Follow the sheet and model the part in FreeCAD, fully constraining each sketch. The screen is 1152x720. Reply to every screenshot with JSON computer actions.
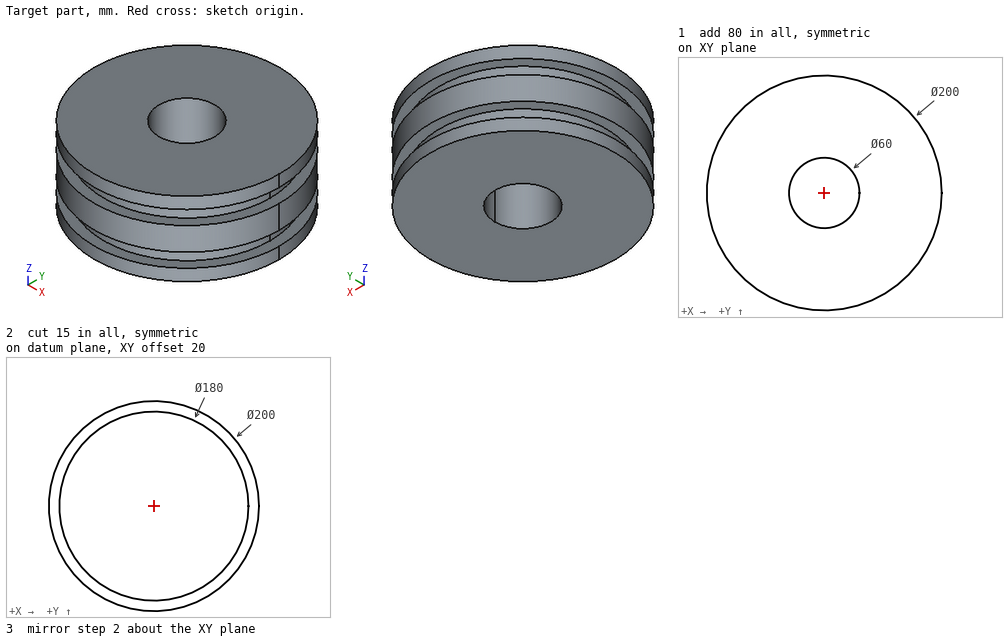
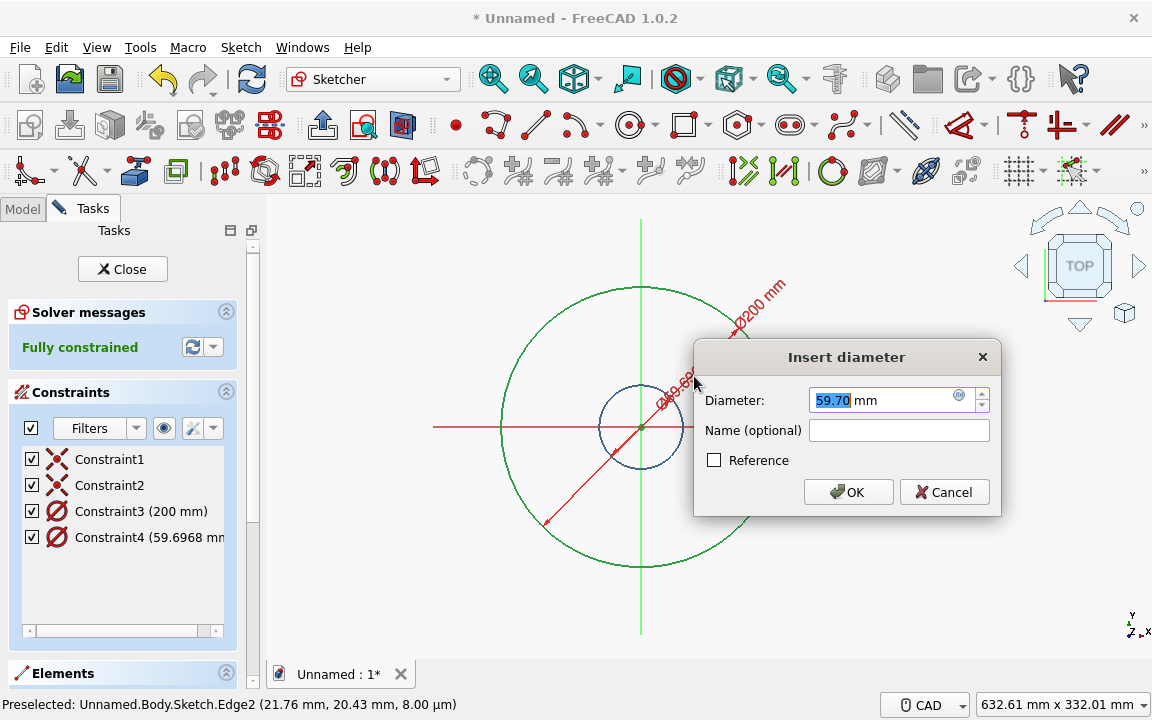
{"action": "type", "text": "60"}
{"action": "key", "text": "Return"}
{"action": "key", "text": "Escape"}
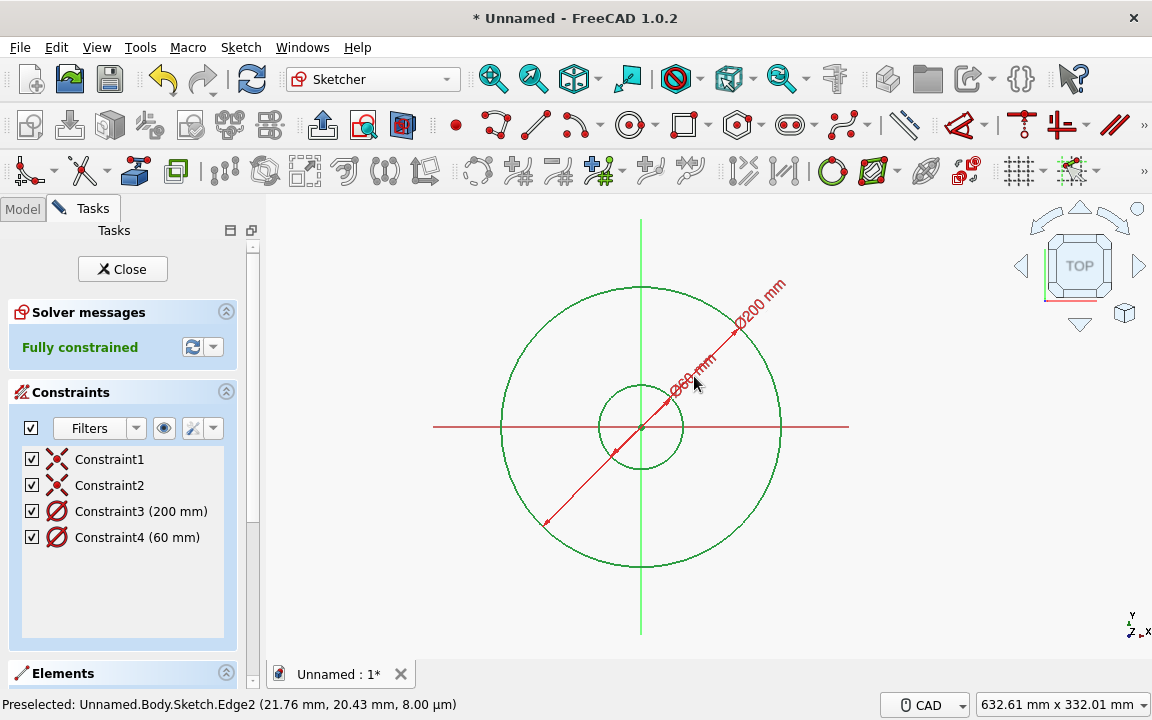
{"action": "left_click", "coordinate": [123, 269]}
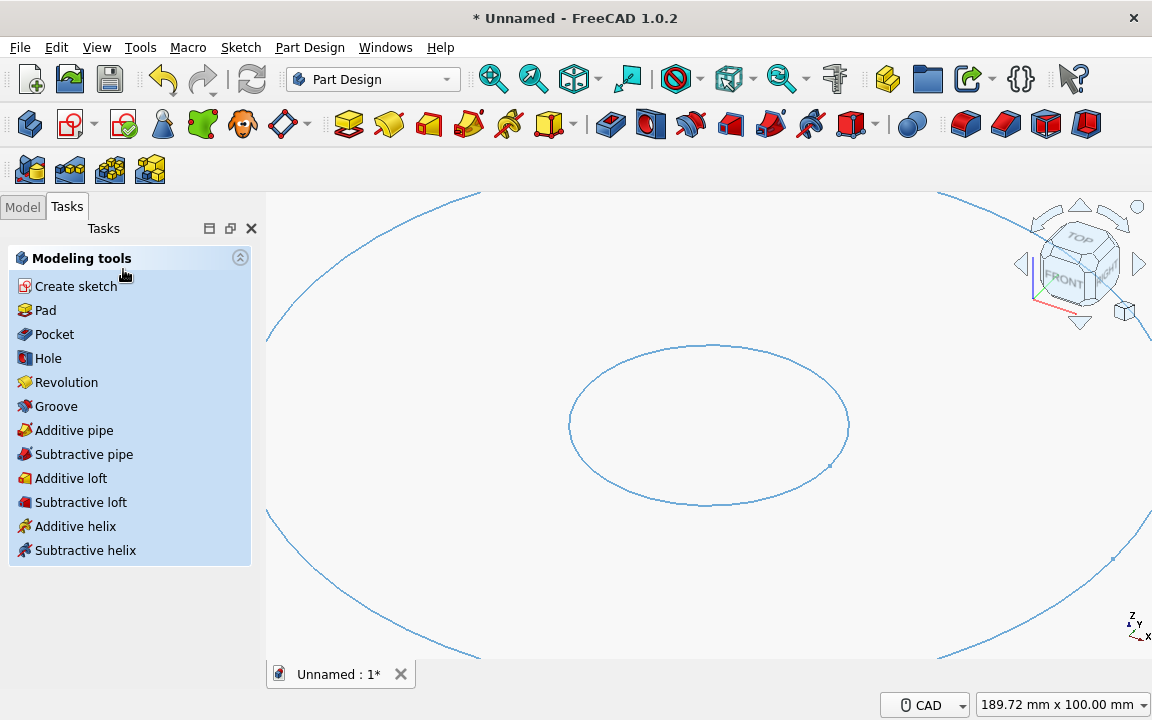
{"action": "left_click", "coordinate": [350, 124]}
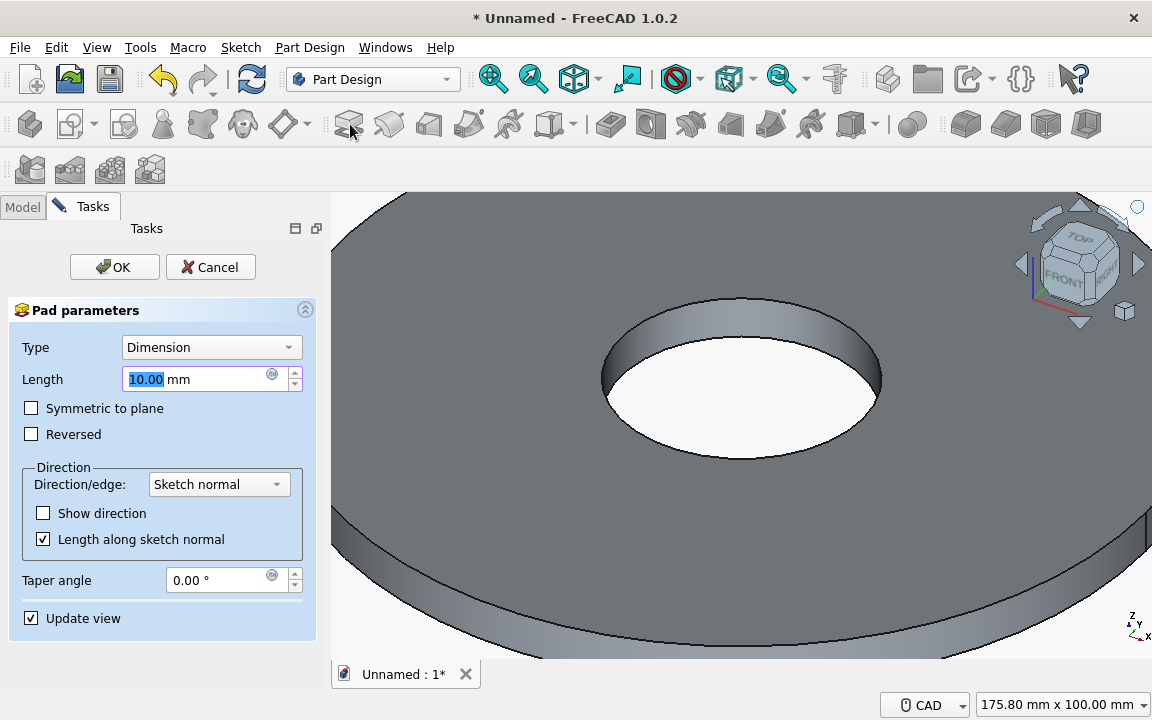
{"action": "type", "text": "80"}
{"action": "key", "text": "Tab"}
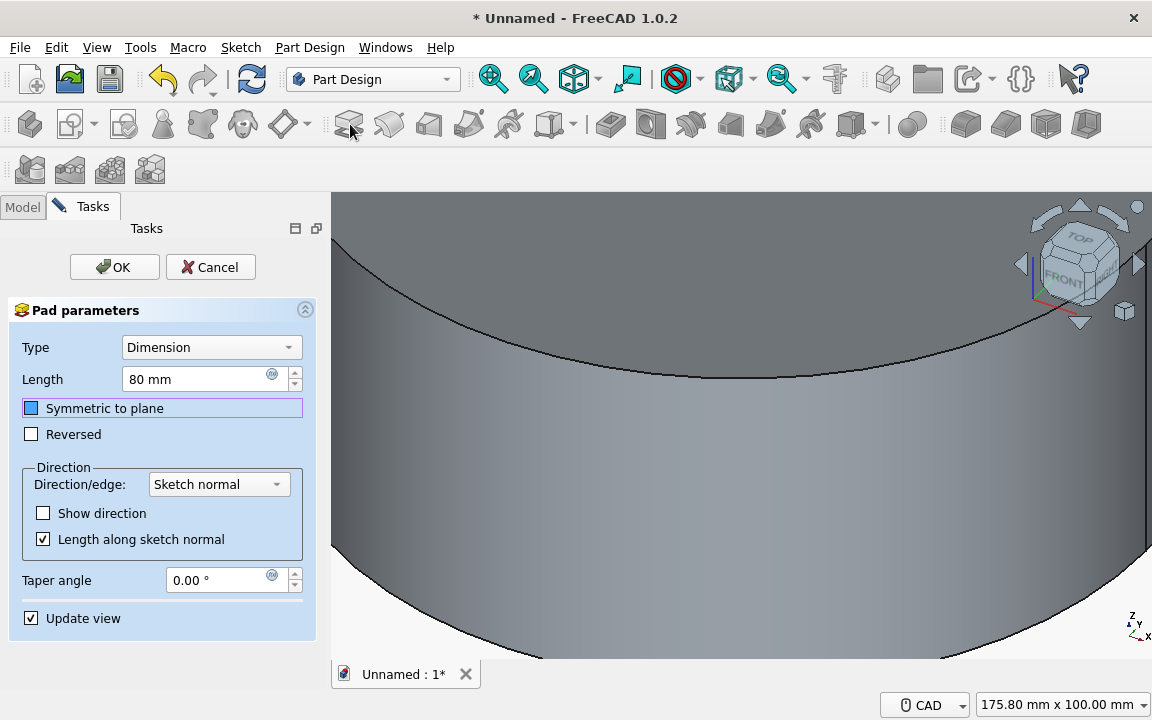
{"action": "left_click", "coordinate": [30, 408]}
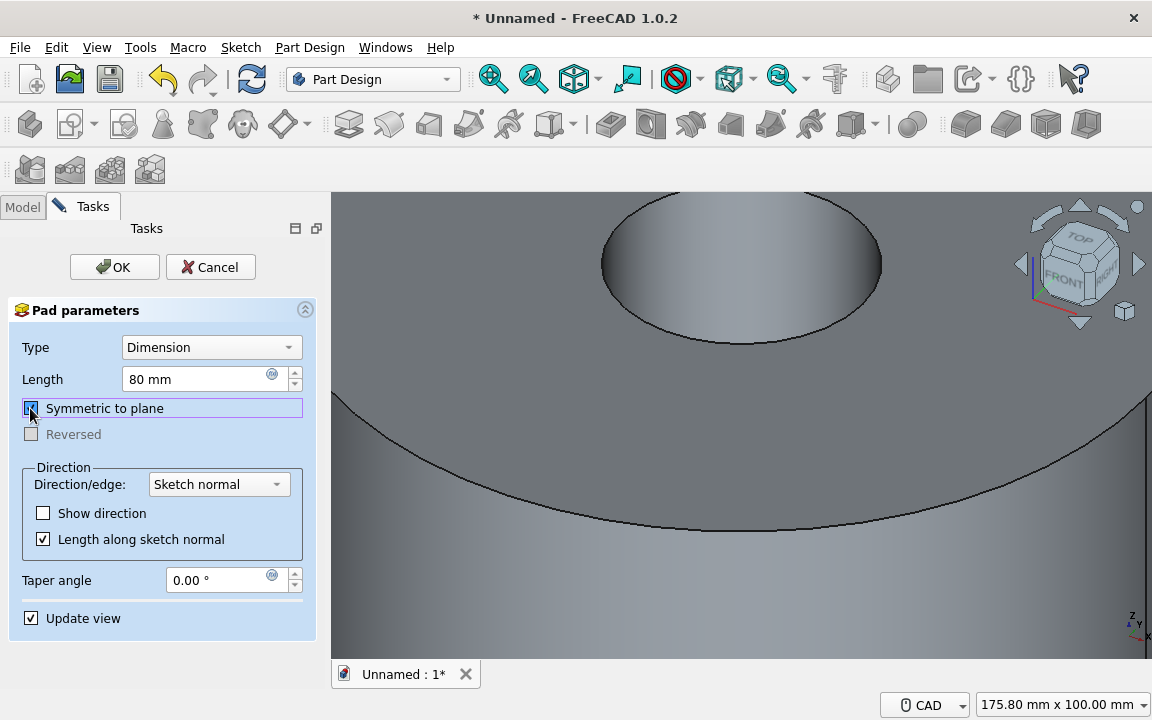
{"action": "left_click", "coordinate": [115, 267]}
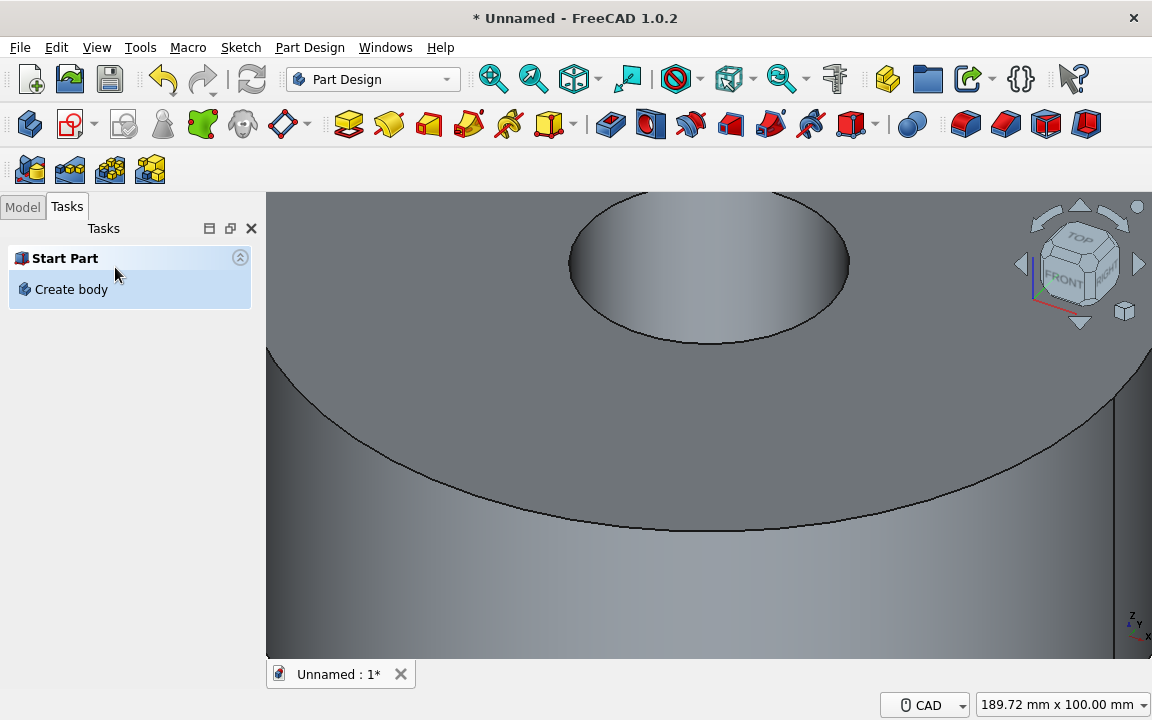
{"action": "left_click", "coordinate": [494, 80]}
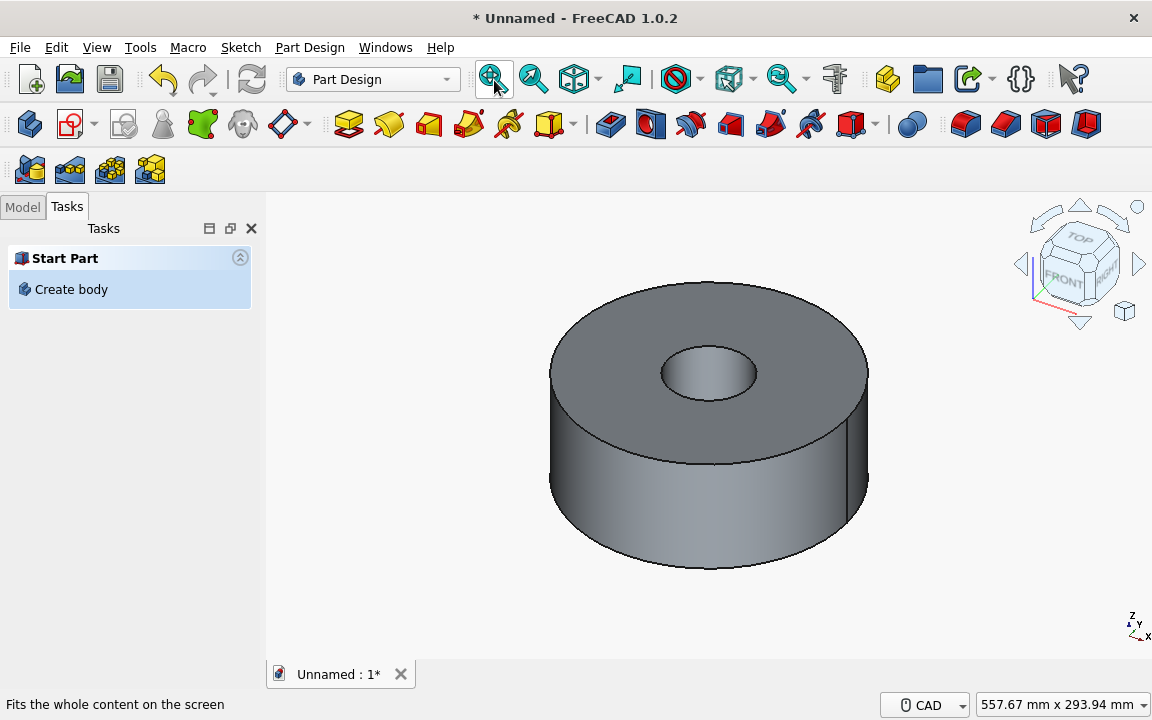
{"action": "left_click", "coordinate": [23, 206]}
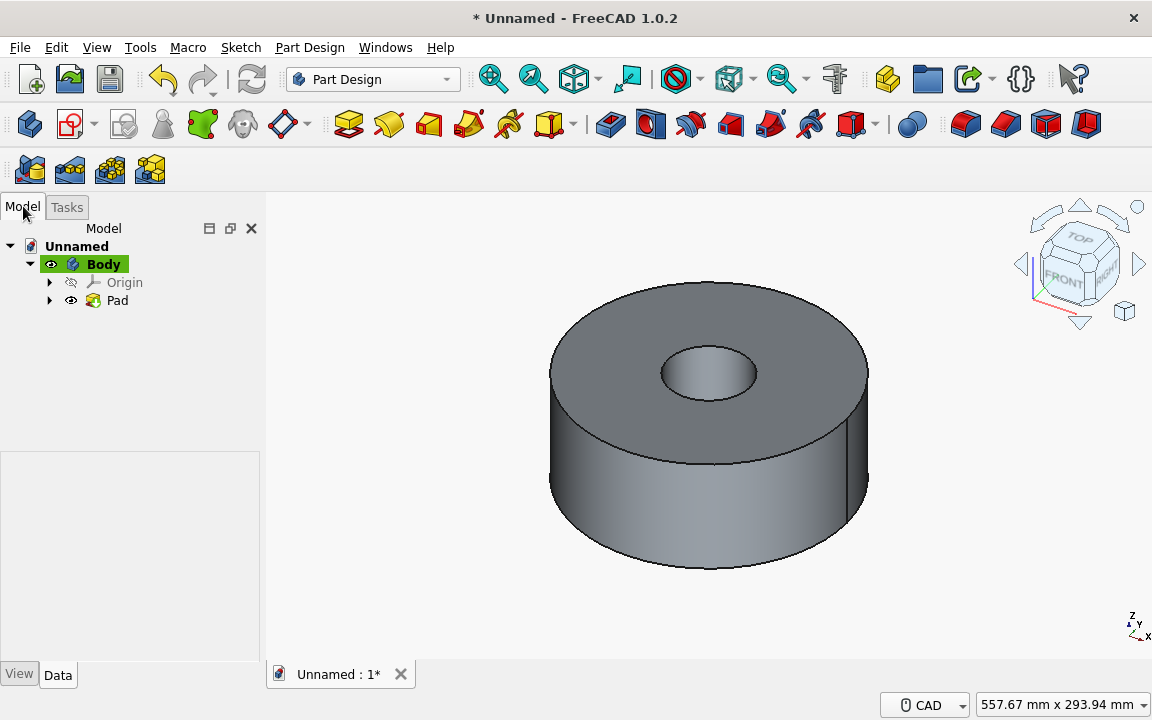
{"action": "left_click", "coordinate": [50, 282]}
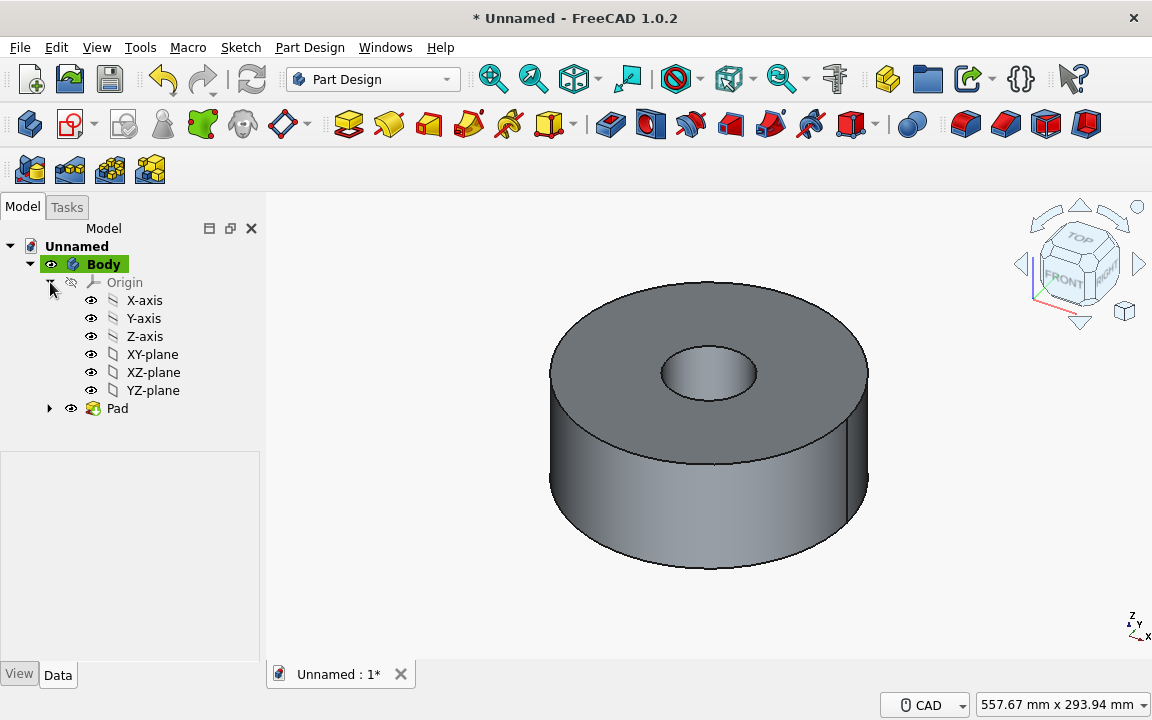
{"action": "left_click", "coordinate": [136, 354]}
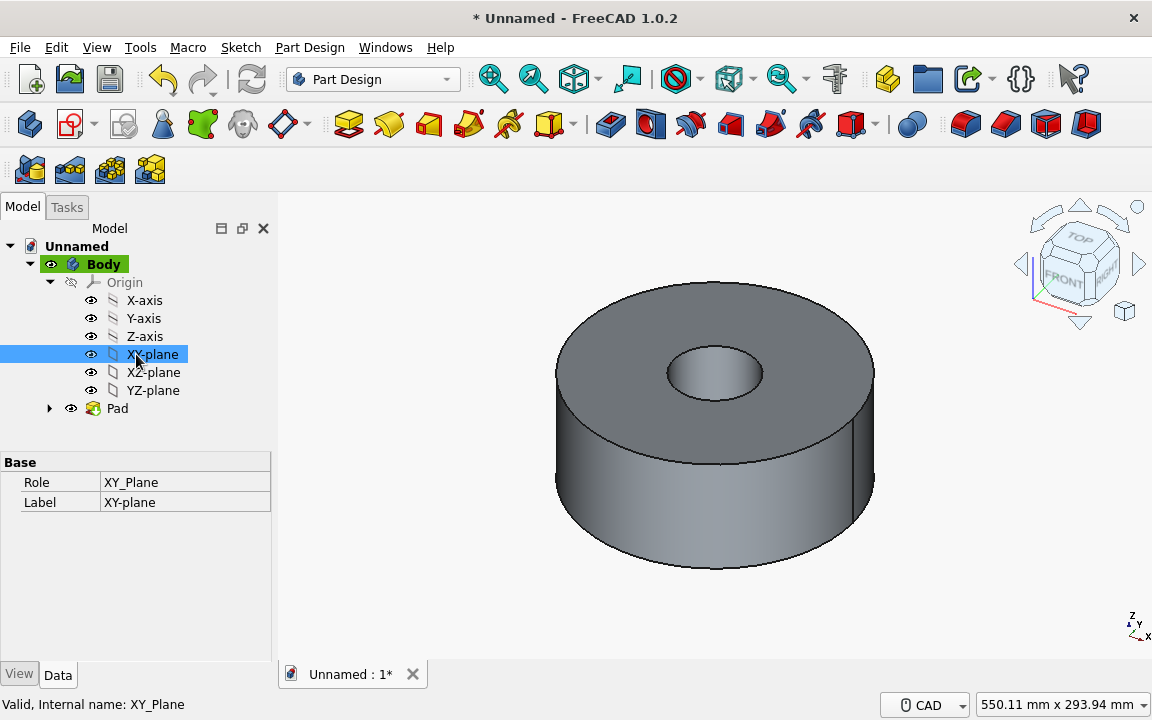
{"action": "left_click", "coordinate": [284, 124]}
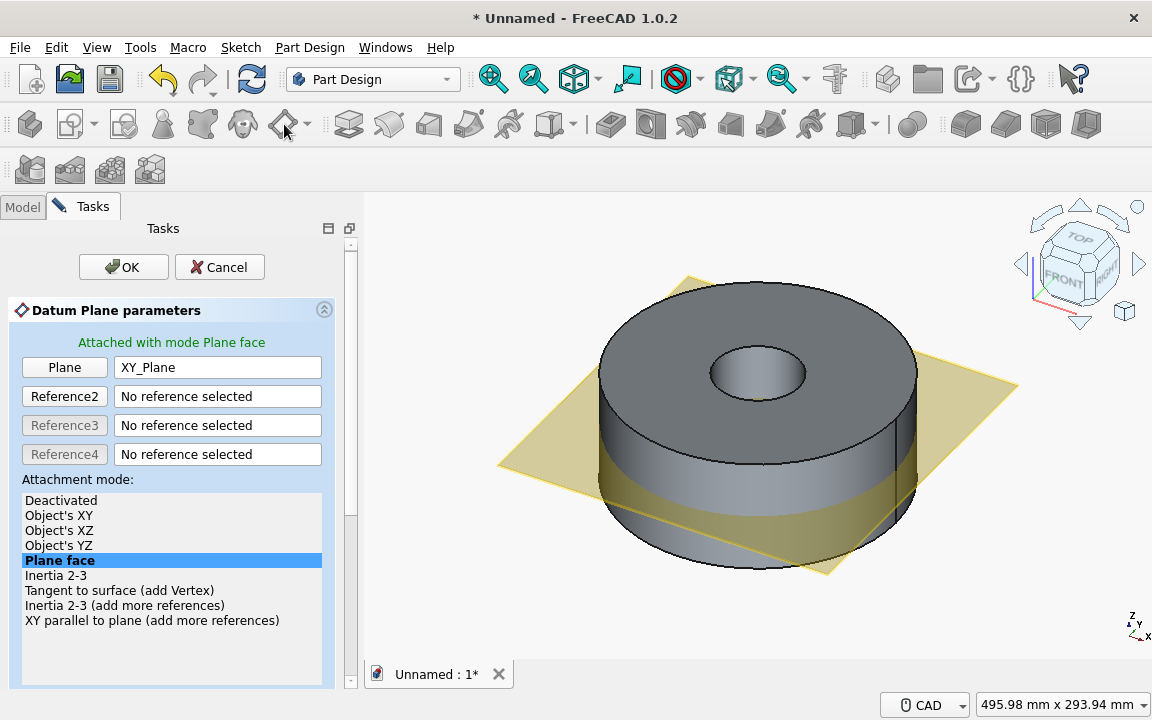
{"action": "scroll", "coordinate": [351, 463], "scroll_direction": "down", "scroll_amount": 3}